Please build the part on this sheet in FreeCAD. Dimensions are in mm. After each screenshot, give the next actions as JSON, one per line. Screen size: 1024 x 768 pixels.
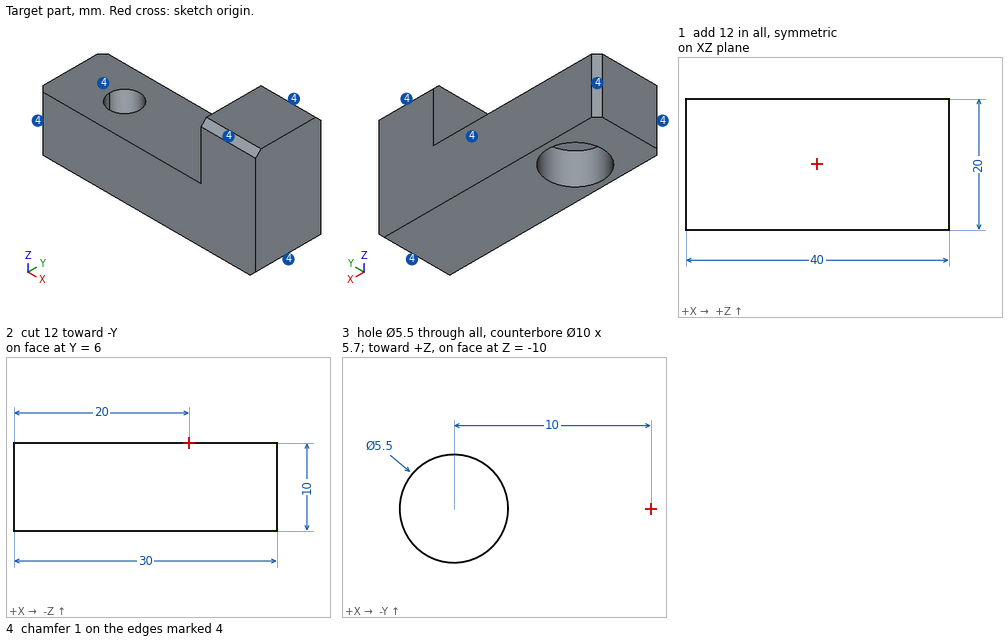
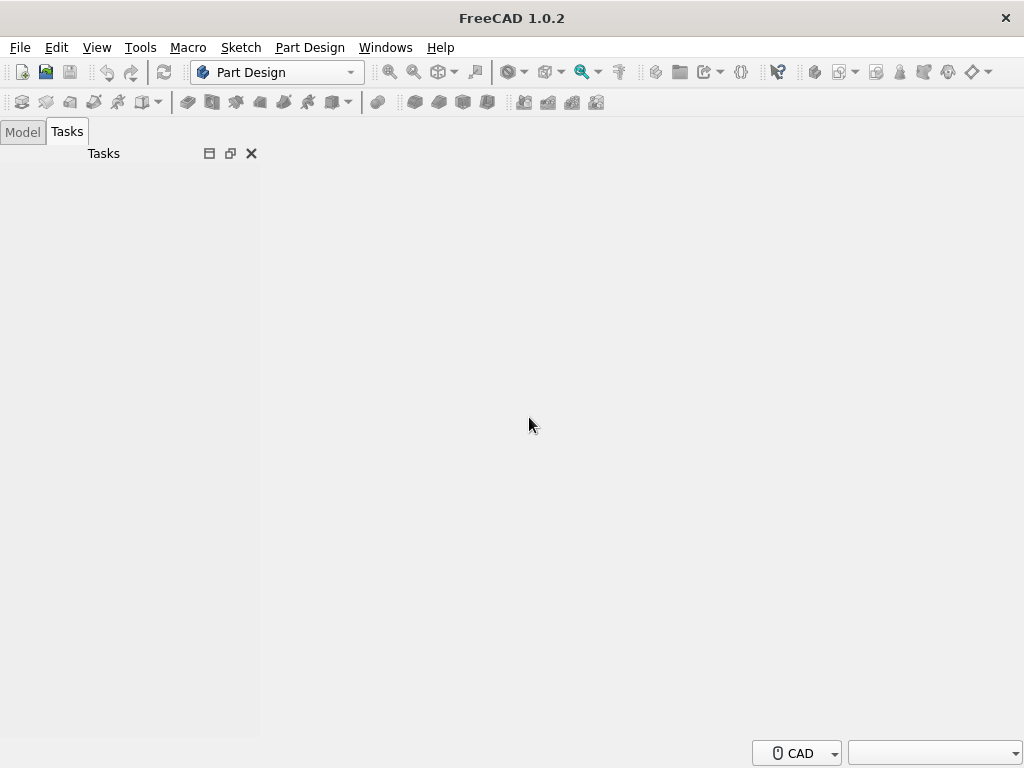
{"action": "key", "text": "ctrl+n"}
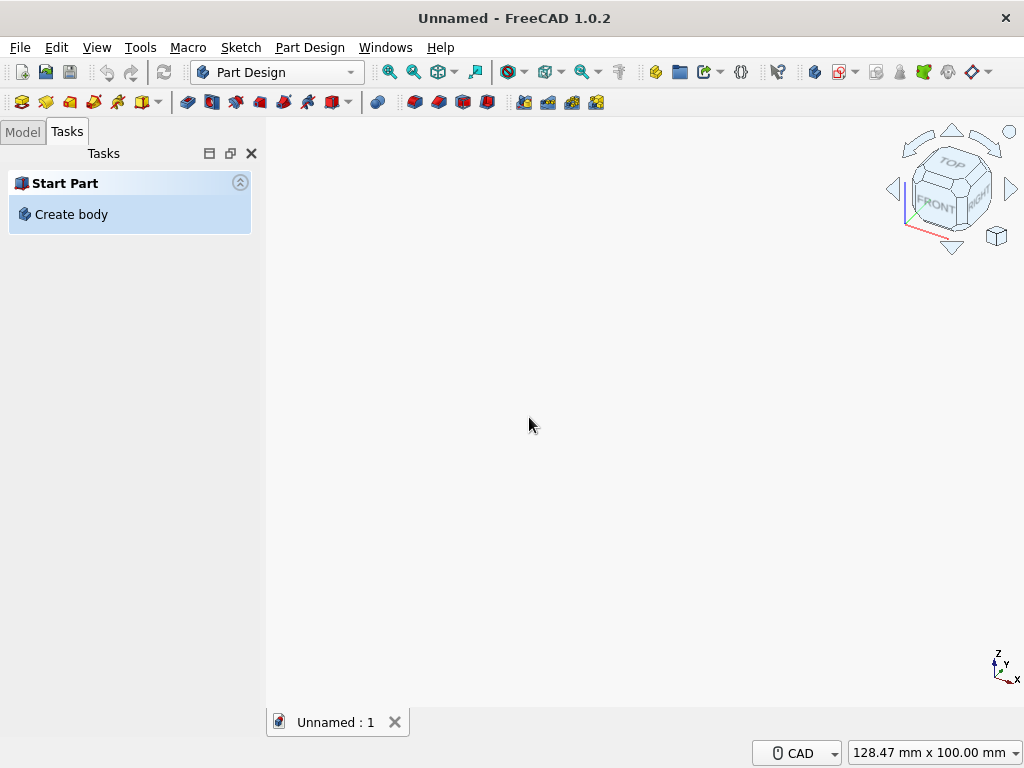
{"action": "left_click", "coordinate": [840, 72]}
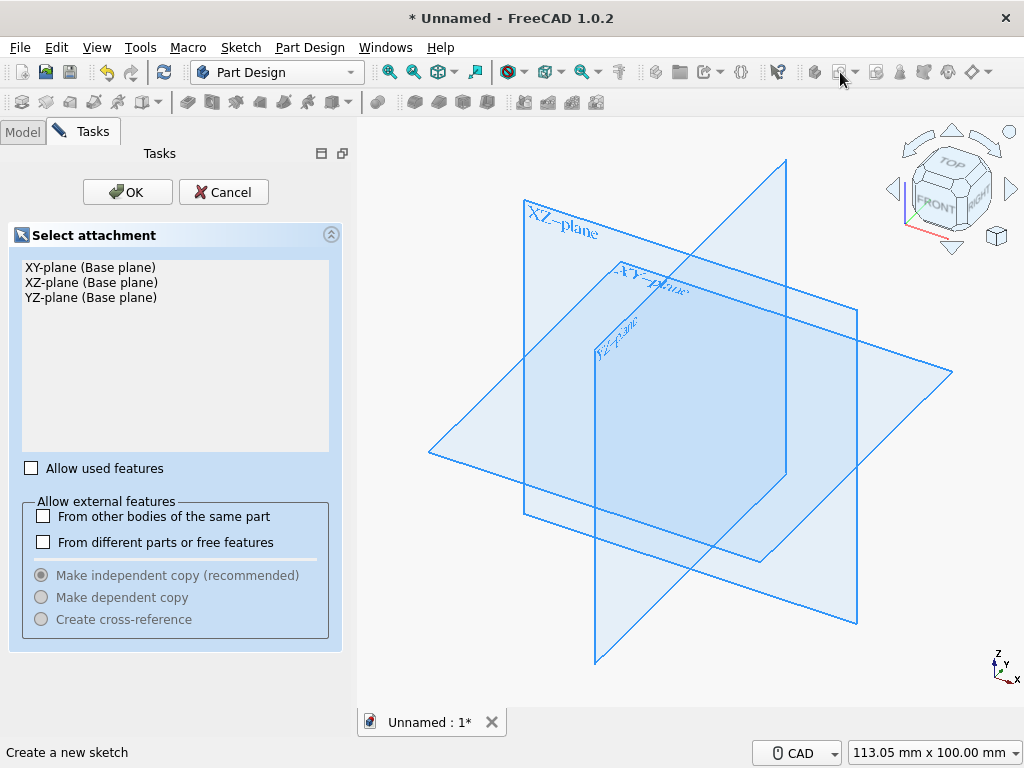
{"action": "left_click", "coordinate": [82, 282]}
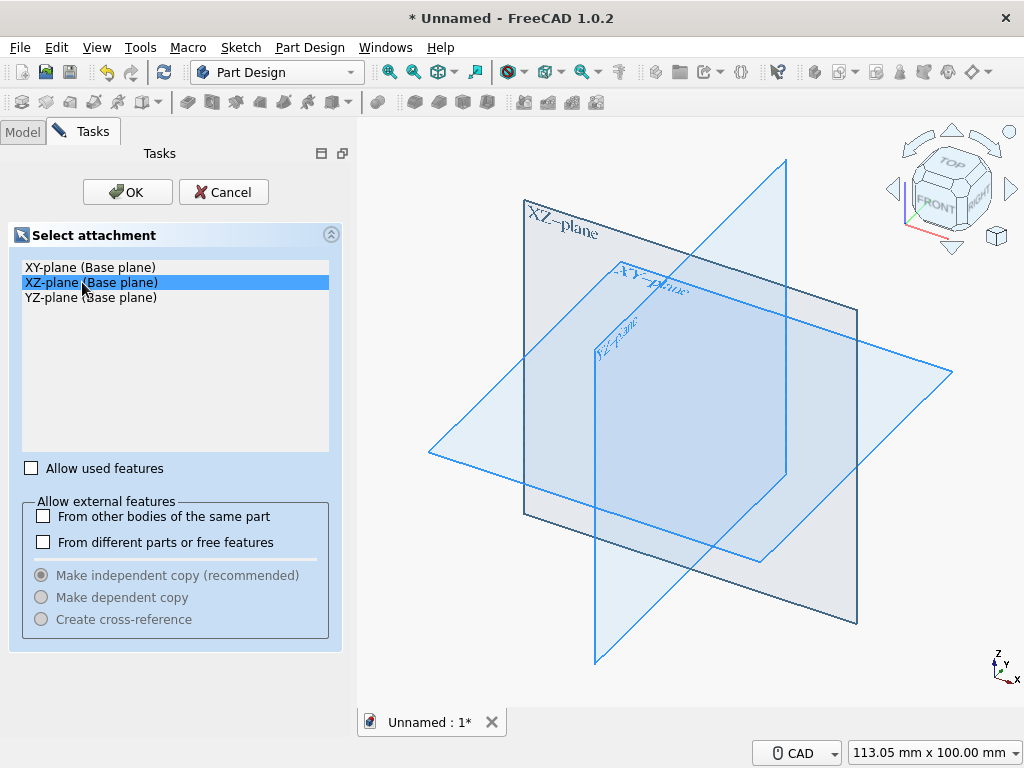
{"action": "left_click", "coordinate": [128, 192]}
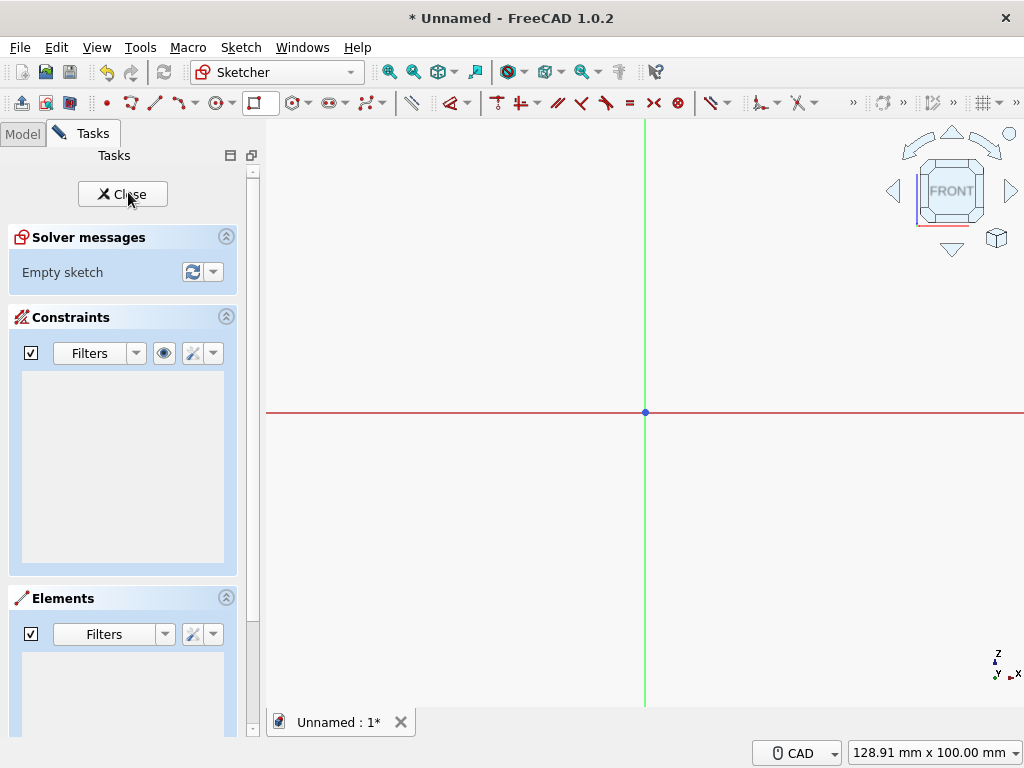
{"action": "scroll", "coordinate": [728, 413], "scroll_direction": "up", "scroll_amount": 3}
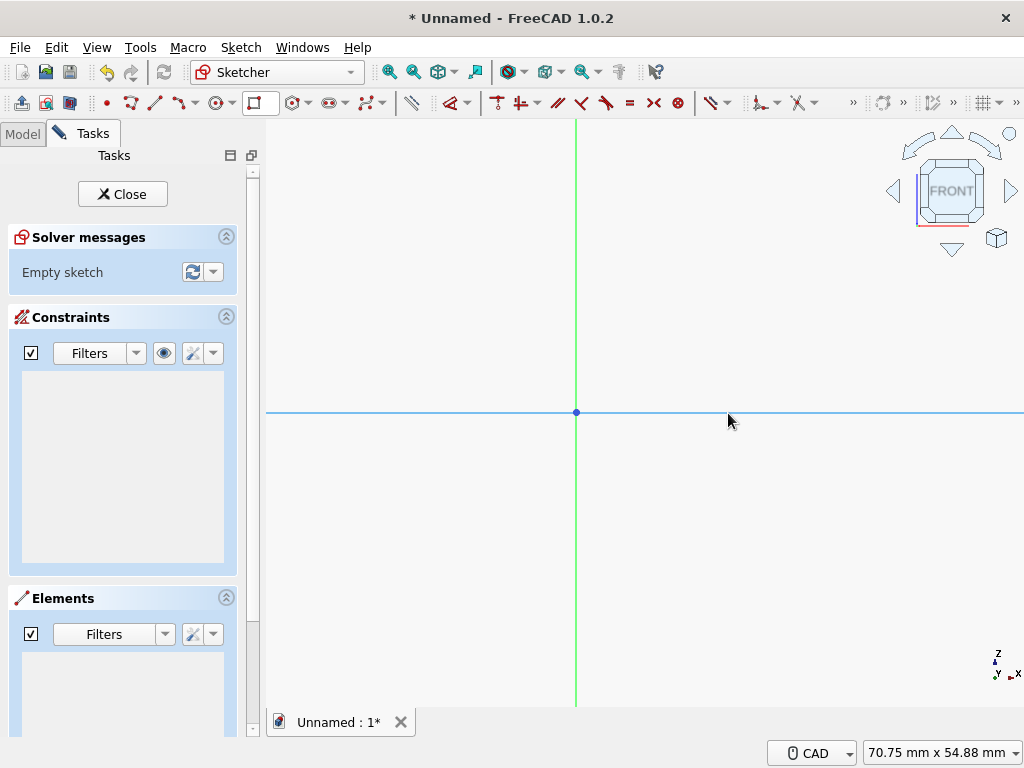
{"action": "key", "text": "g v"}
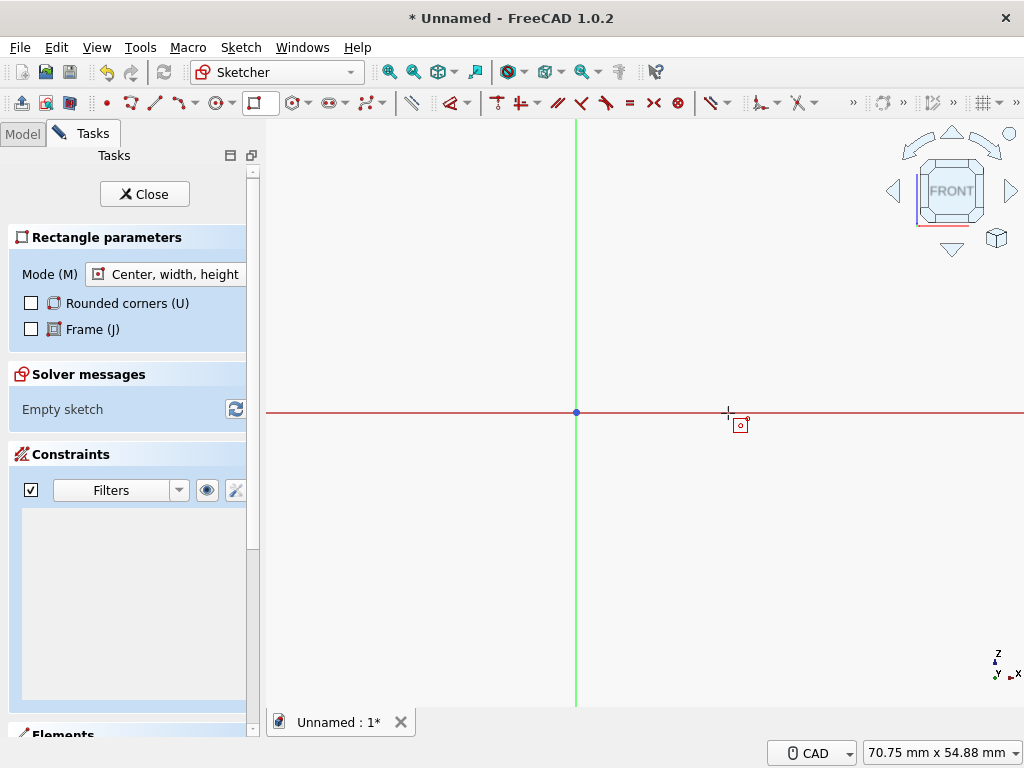
{"action": "left_click", "coordinate": [576, 413]}
{"action": "mouse_move", "coordinate": [791, 305]}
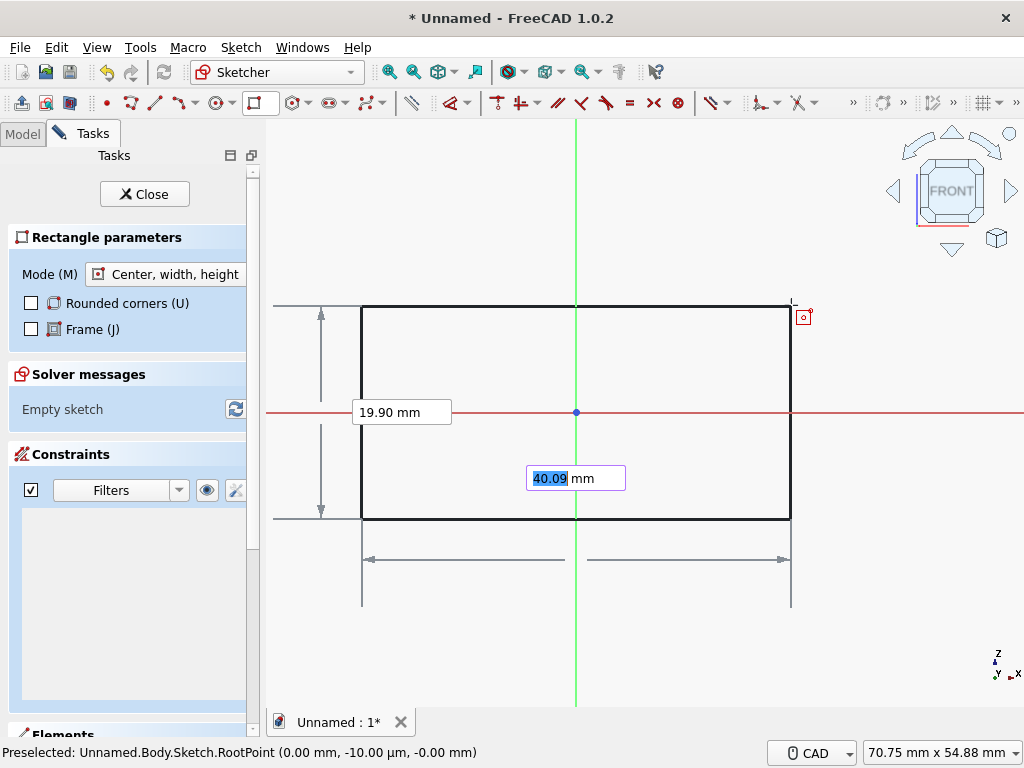
{"action": "type", "text": "40"}
{"action": "key", "text": "Tab"}
{"action": "type", "text": "20"}
{"action": "key", "text": "Return"}
{"action": "key", "text": "Escape"}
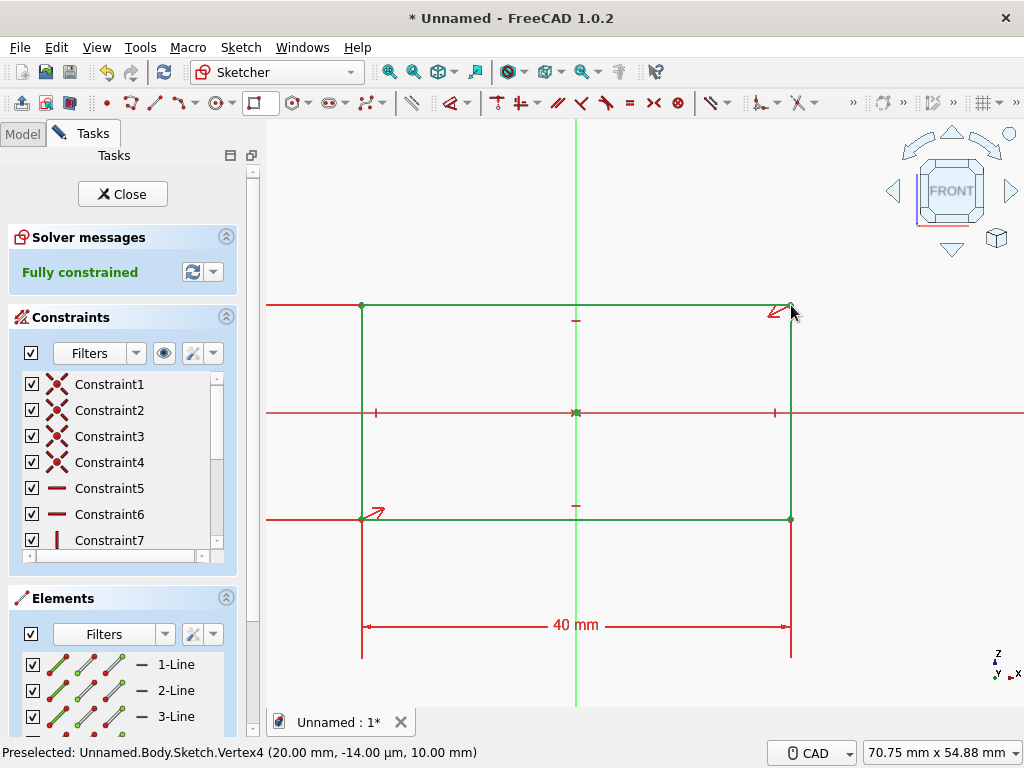
{"action": "left_click", "coordinate": [123, 194]}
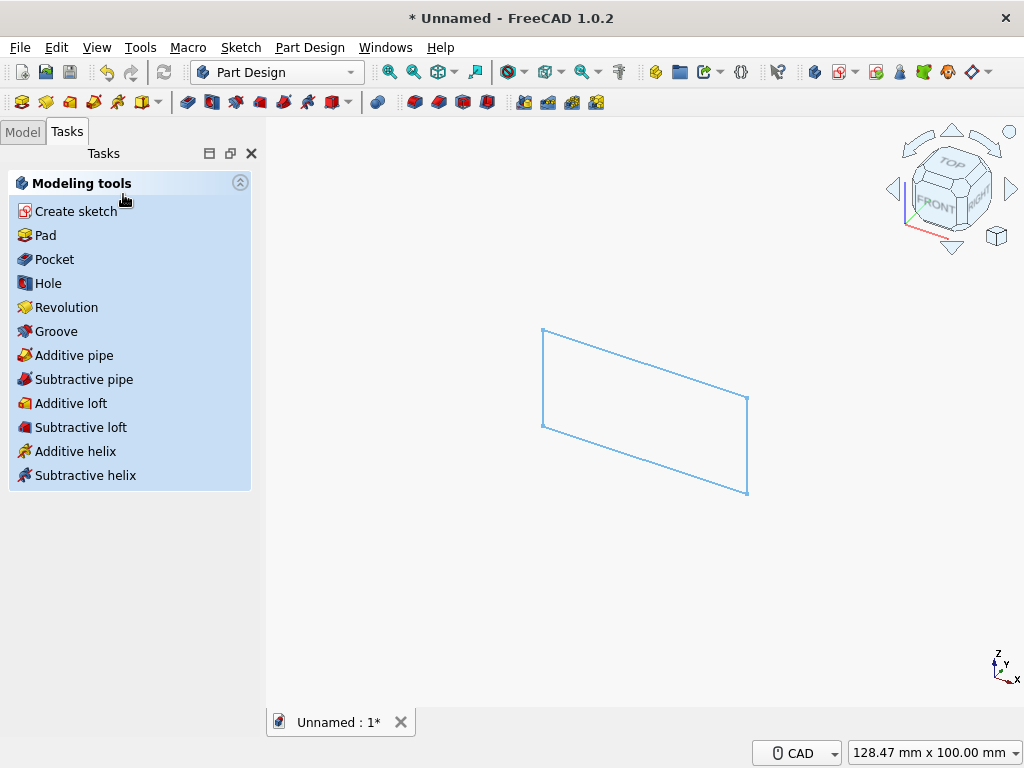
{"action": "left_click", "coordinate": [22, 102]}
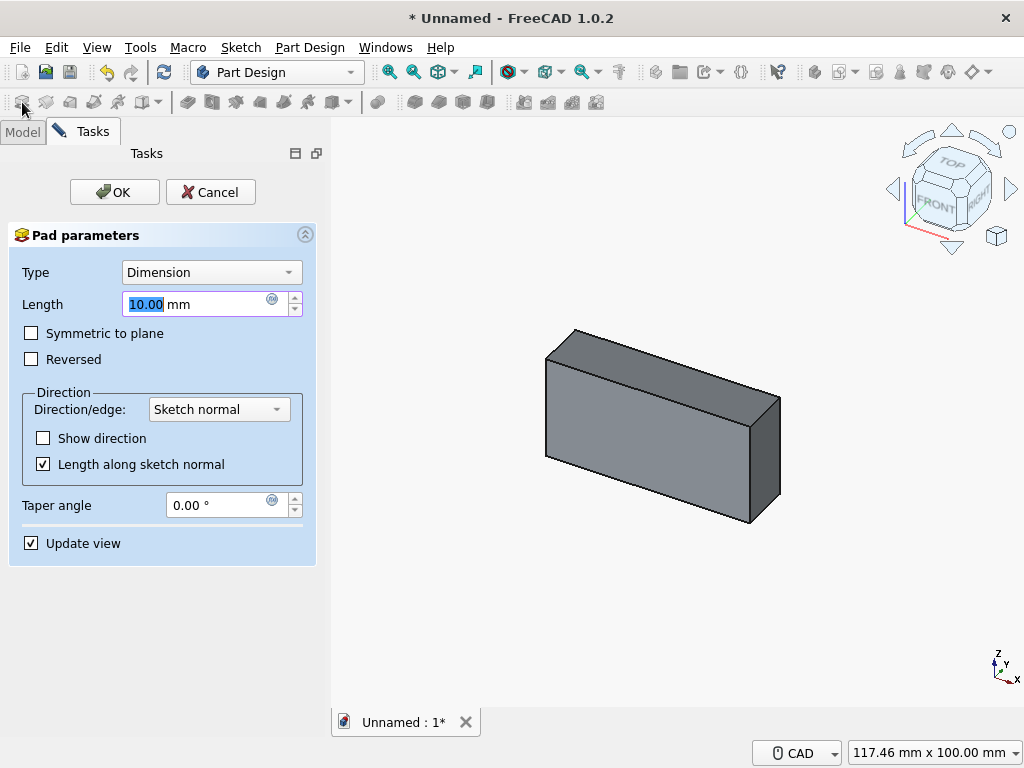
{"action": "type", "text": "12"}
{"action": "key", "text": "Tab"}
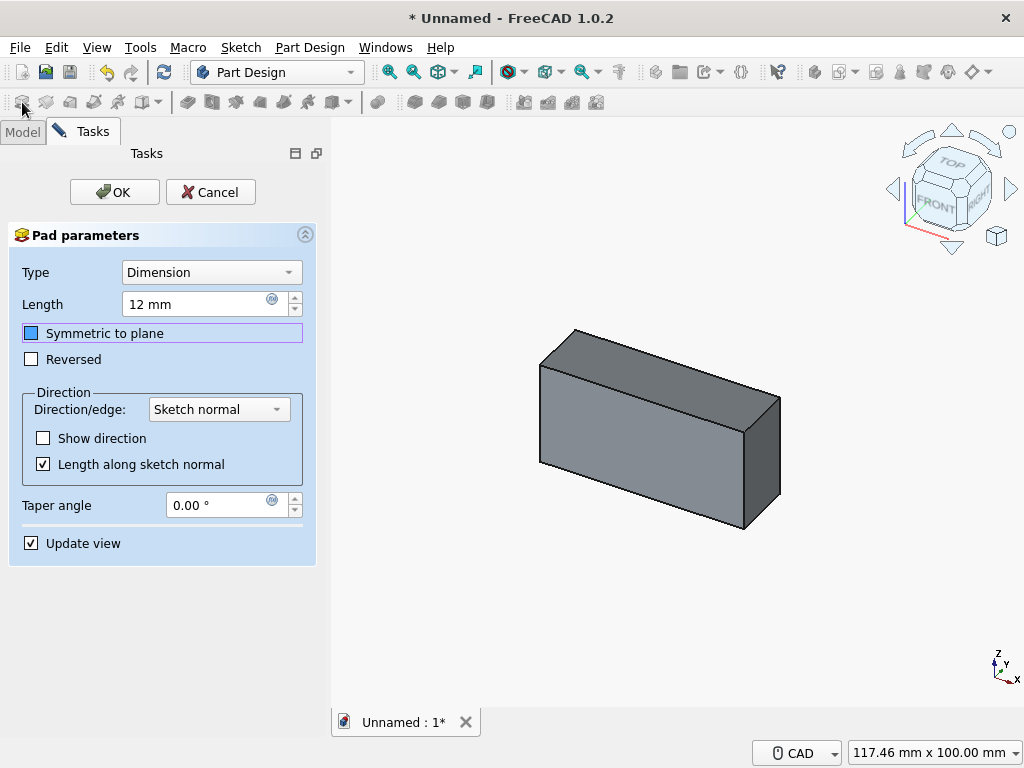
{"action": "left_click", "coordinate": [30, 333]}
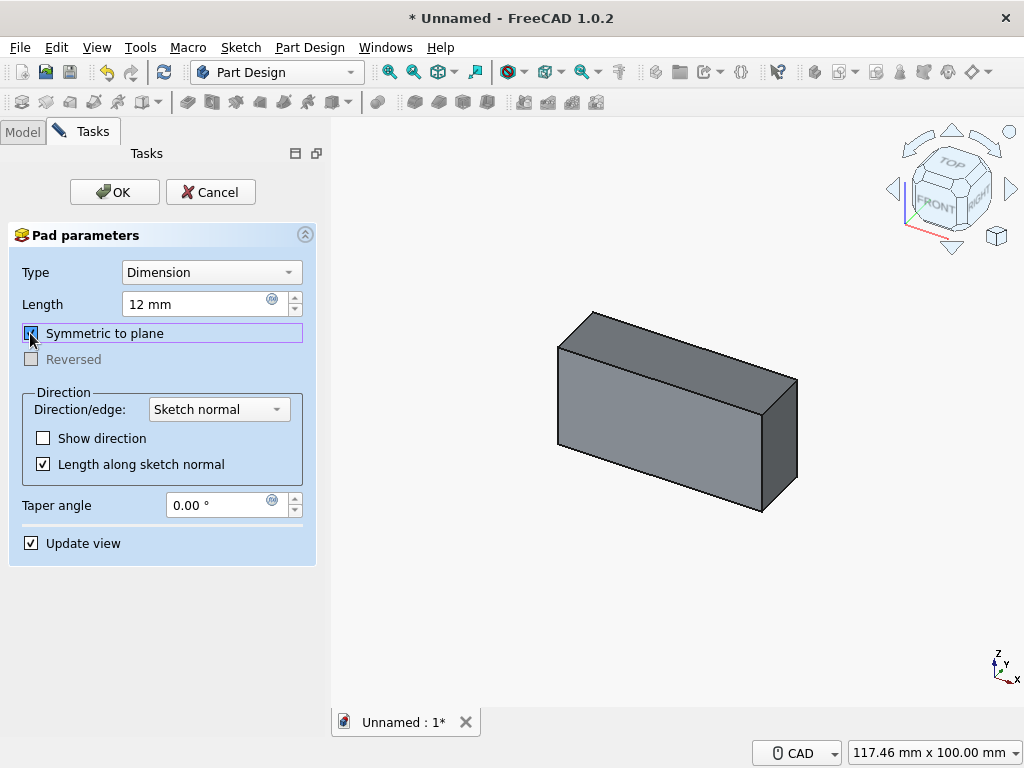
{"action": "left_click", "coordinate": [115, 192]}